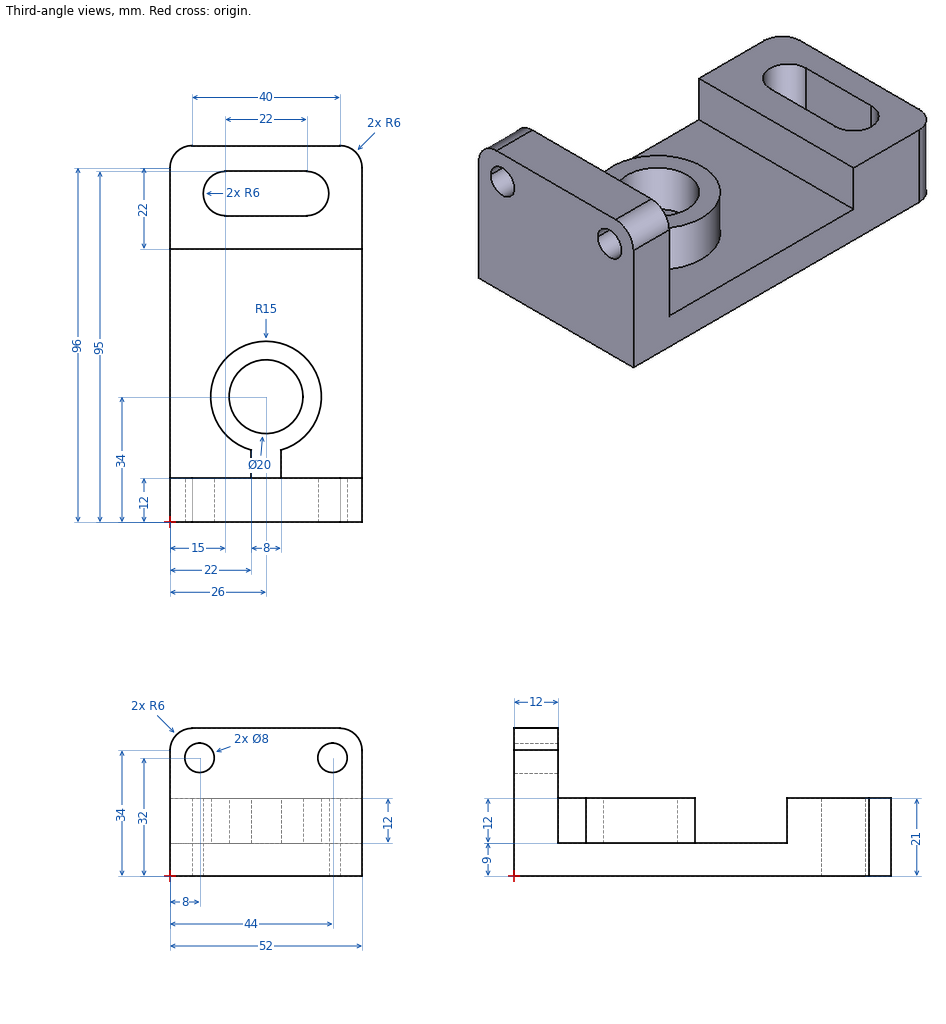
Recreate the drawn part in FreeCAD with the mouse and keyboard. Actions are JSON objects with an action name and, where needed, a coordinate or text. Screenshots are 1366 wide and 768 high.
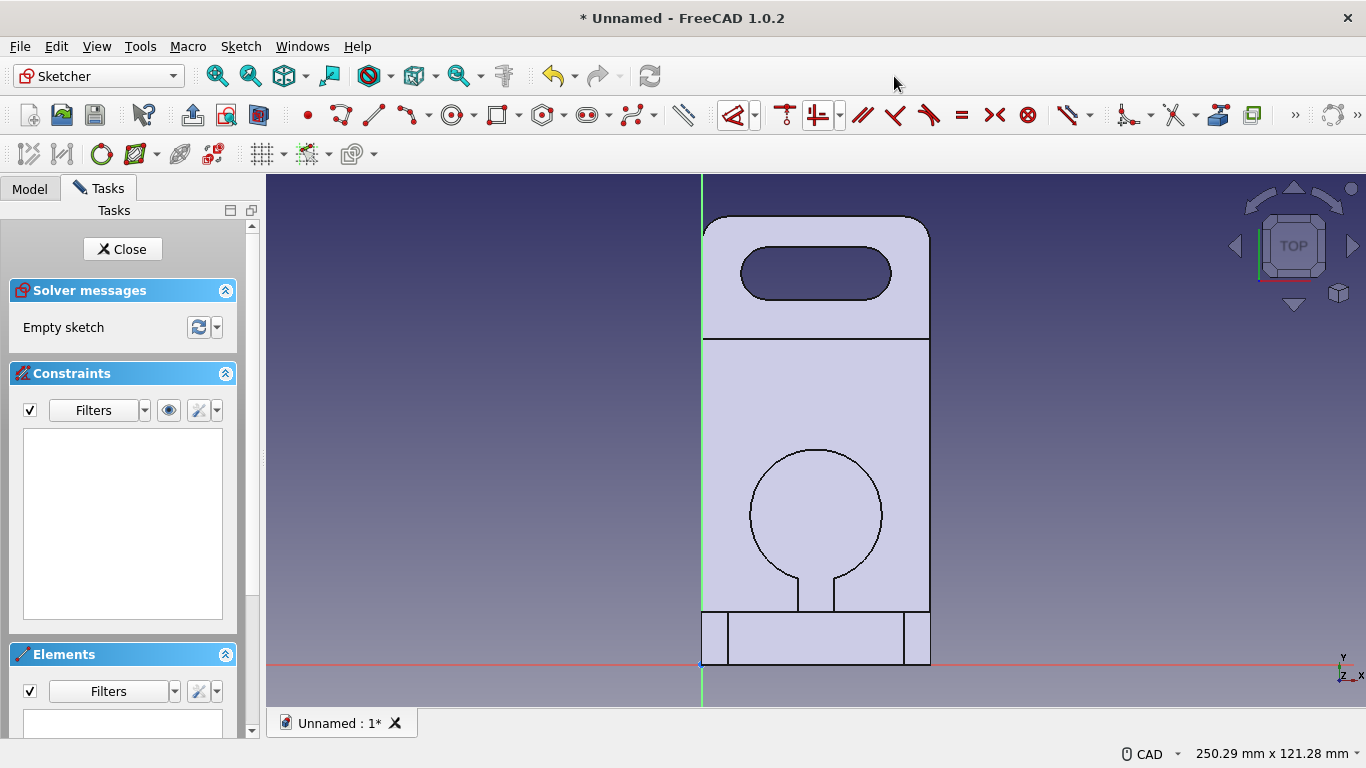
{"action": "left_click", "coordinate": [259, 116]}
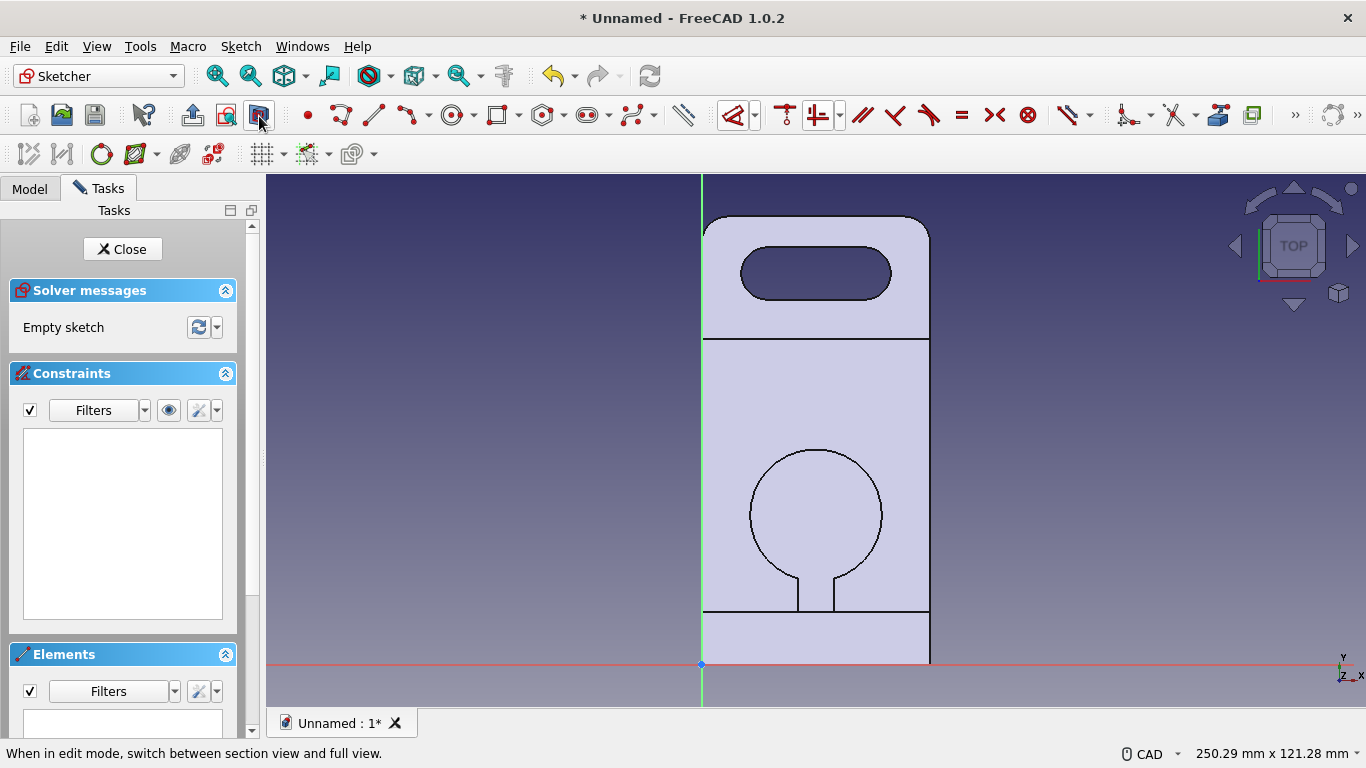
{"action": "scroll", "coordinate": [821, 679], "scroll_direction": "up", "scroll_amount": 3}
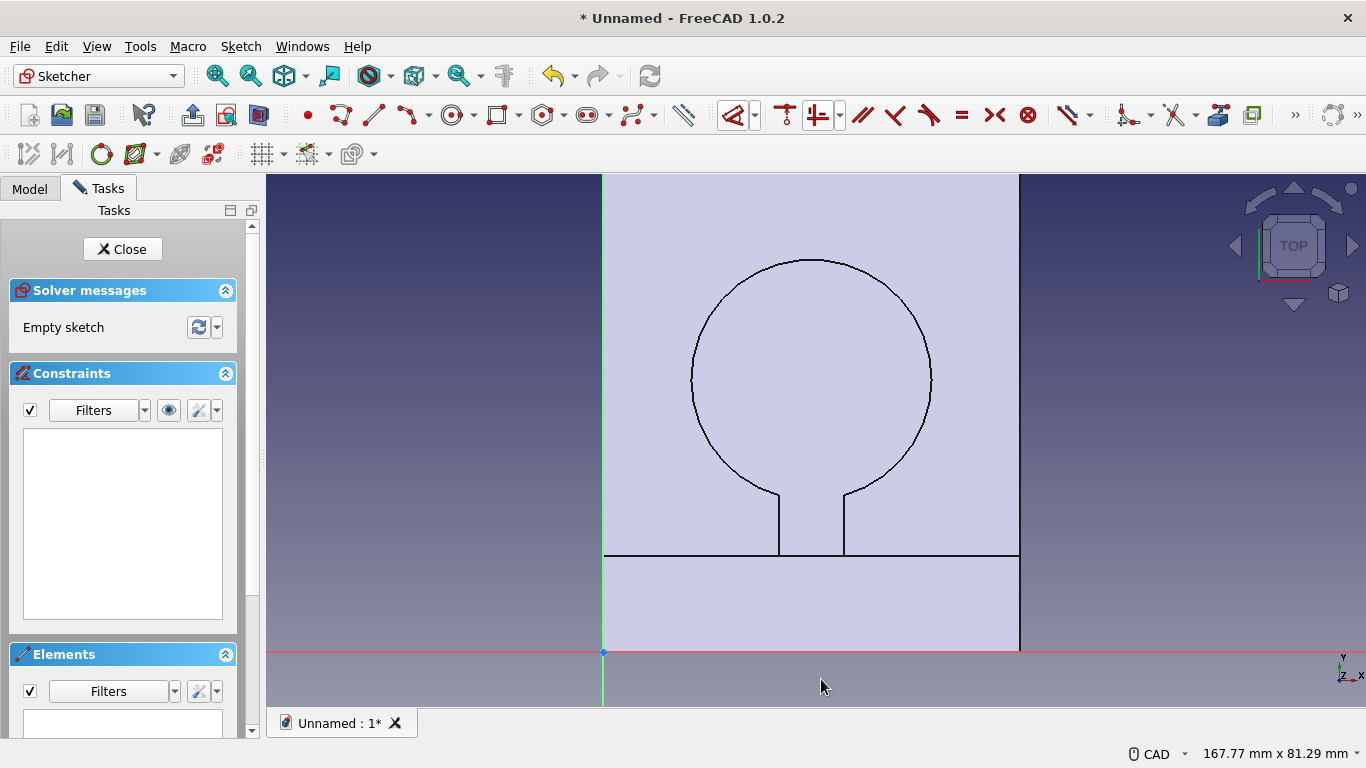
{"action": "left_click", "coordinate": [452, 116]}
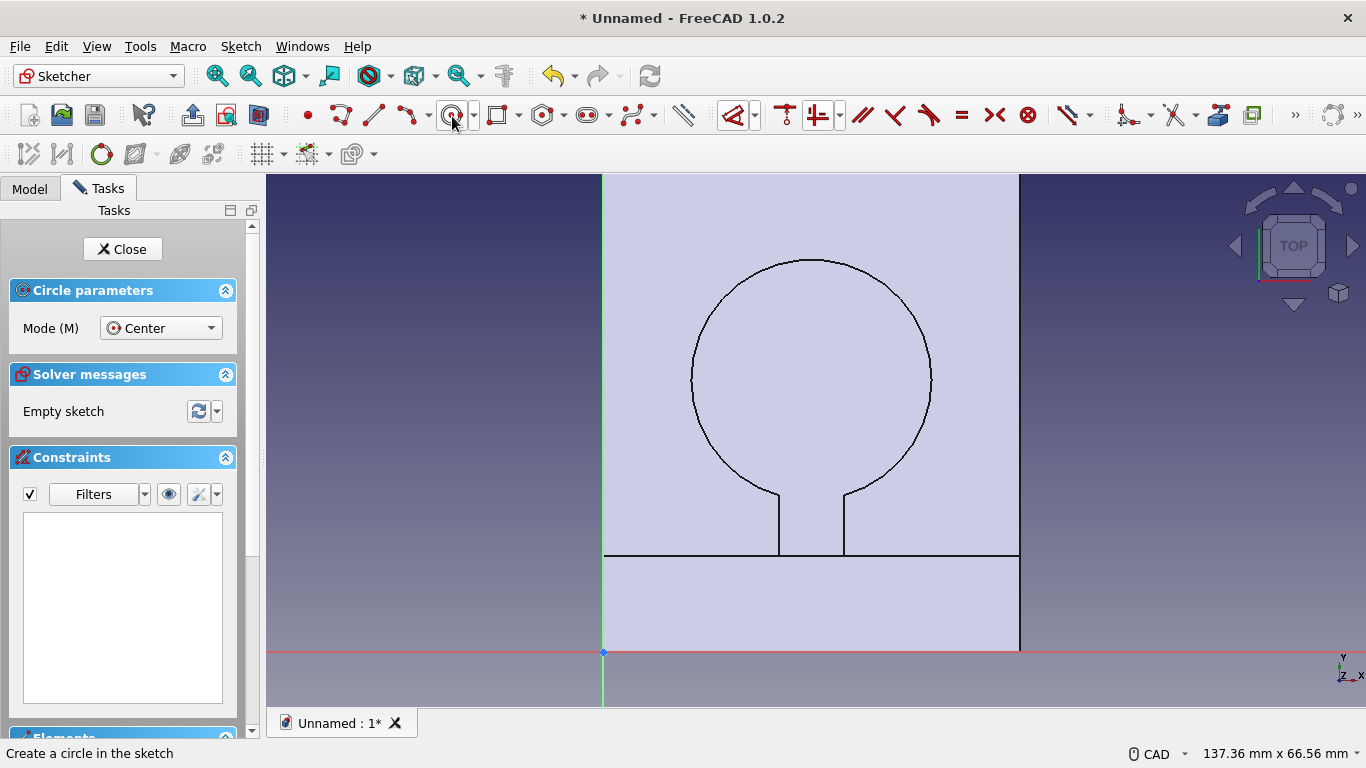
{"action": "left_click", "coordinate": [811, 380]}
{"action": "mouse_move", "coordinate": [868, 323]}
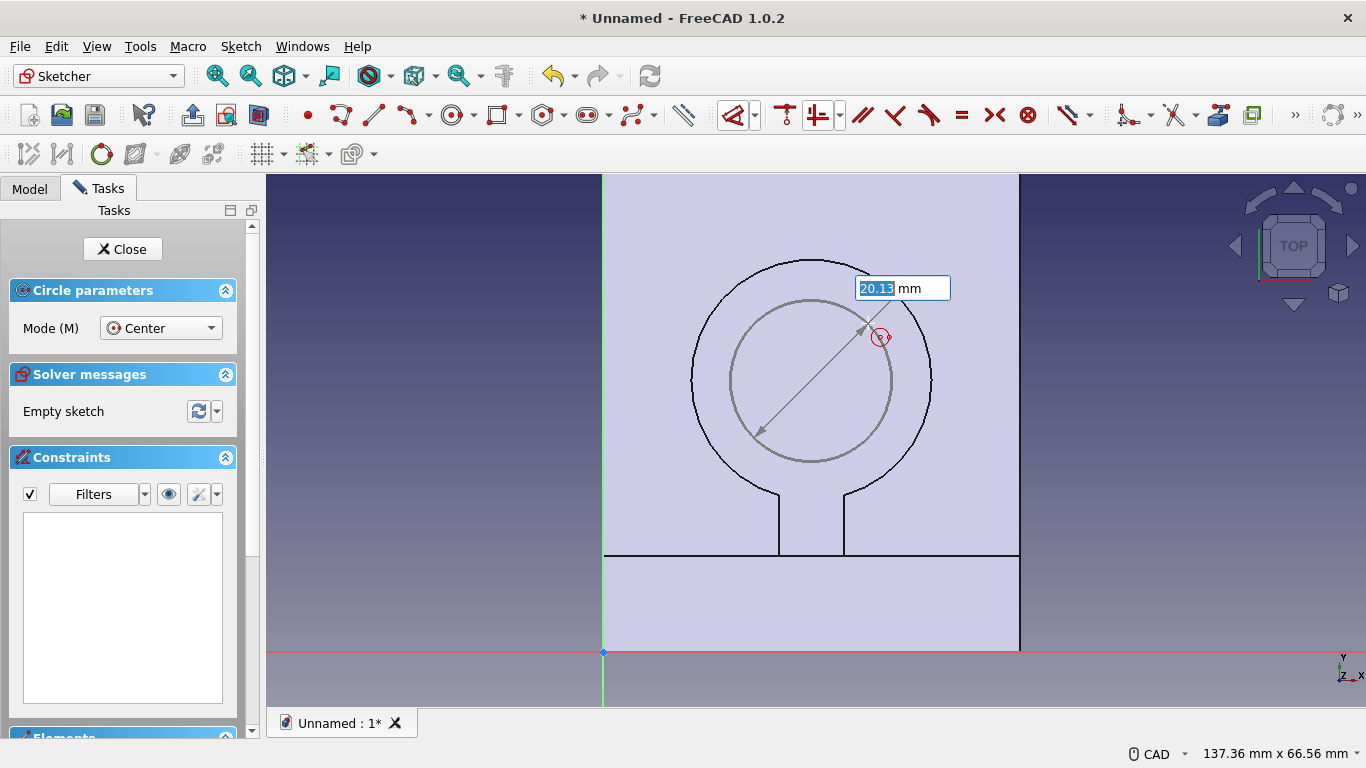
{"action": "type", "text": "20"}
{"action": "key", "text": "Return"}
{"action": "key", "text": "Escape"}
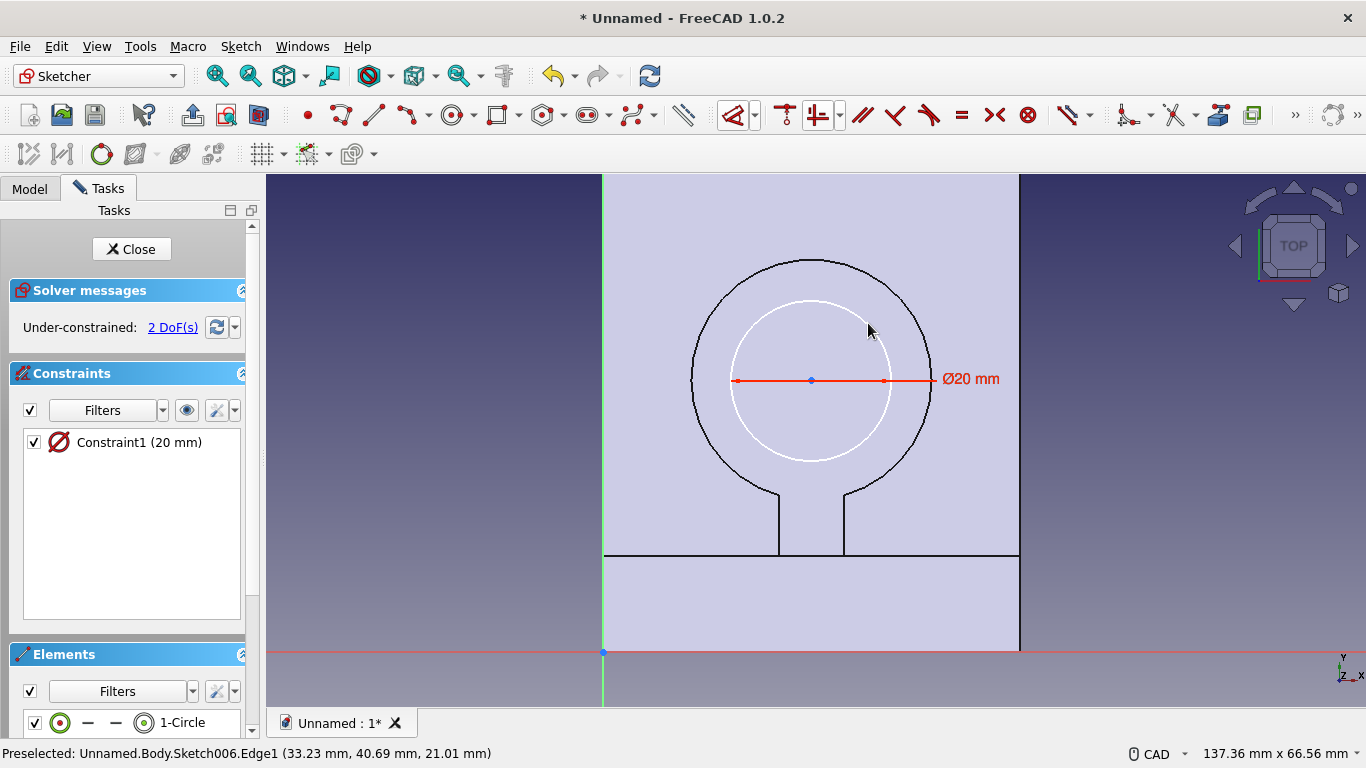
{"action": "left_click", "coordinate": [811, 381]}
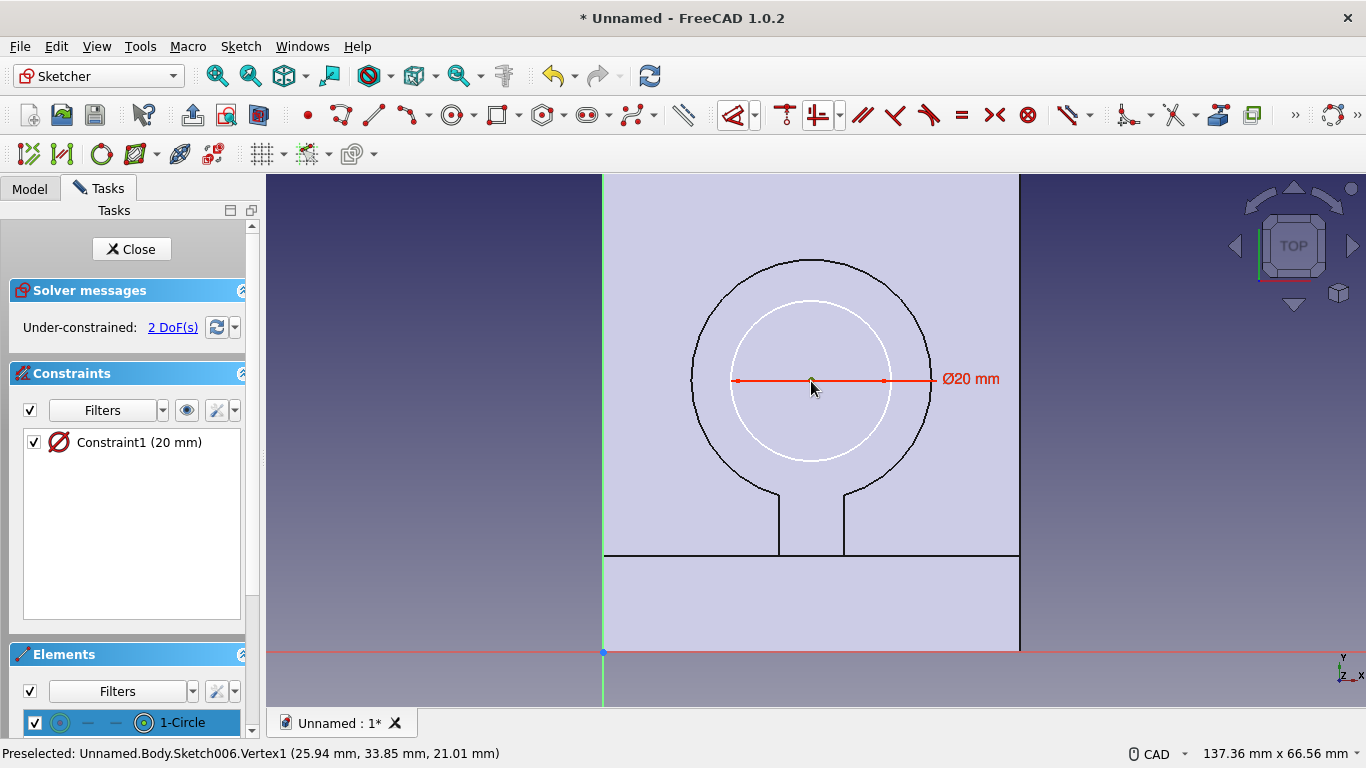
{"action": "left_click", "coordinate": [754, 116]}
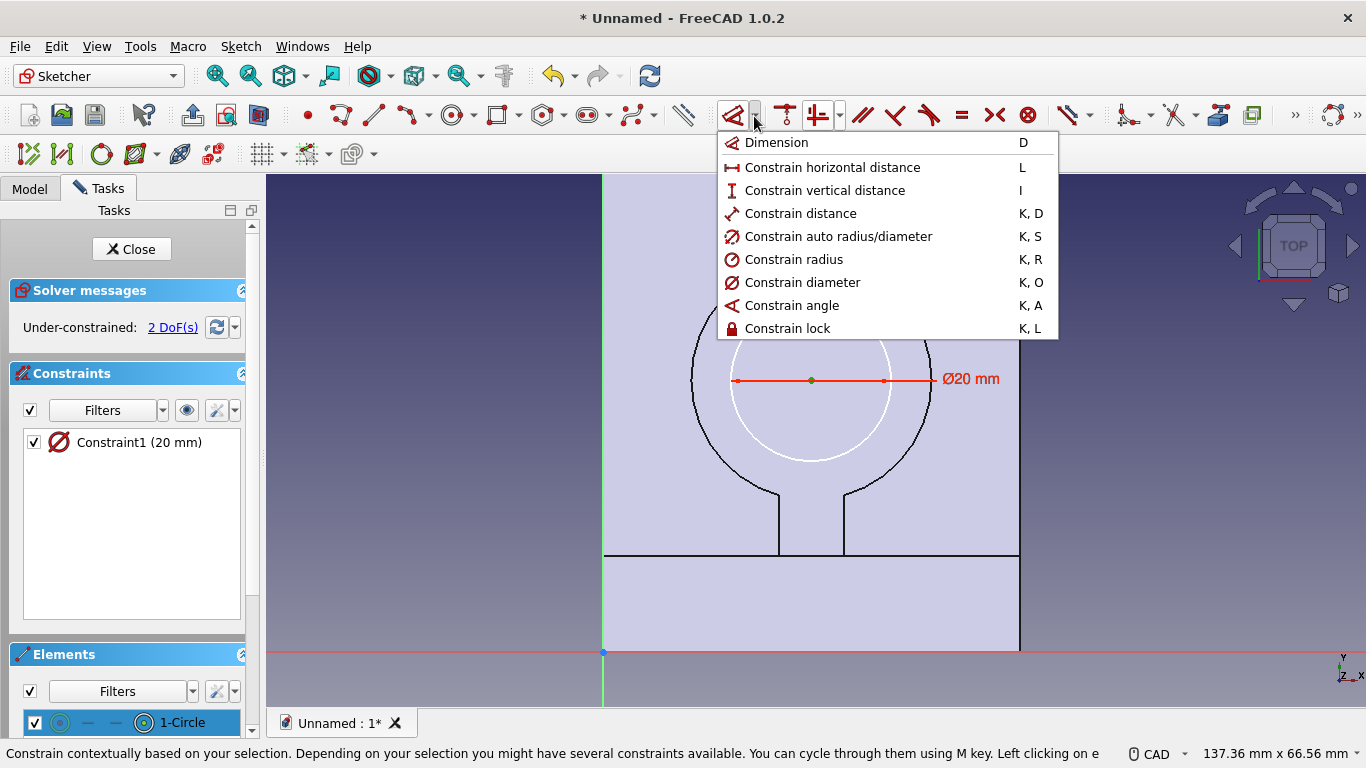
{"action": "left_click", "coordinate": [888, 168]}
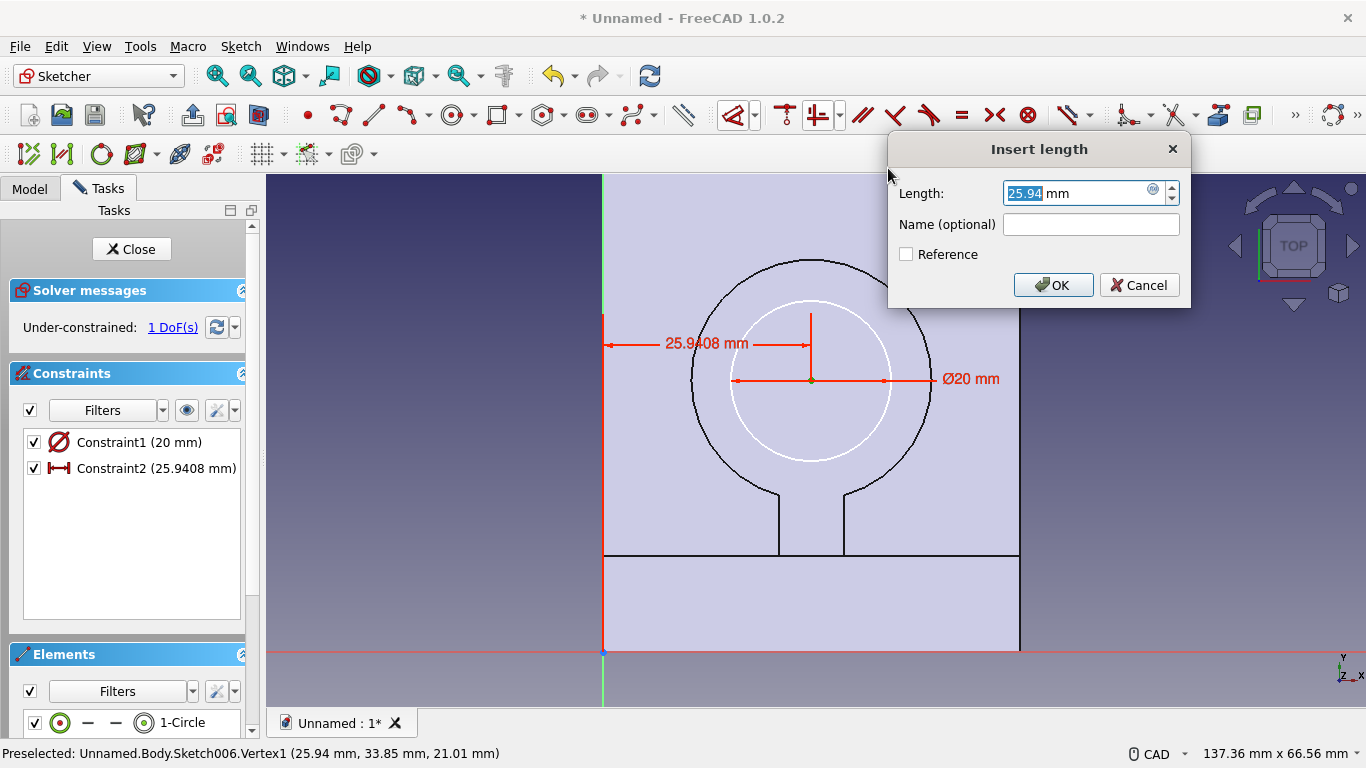
{"action": "type", "text": "26"}
{"action": "key", "text": "Return"}